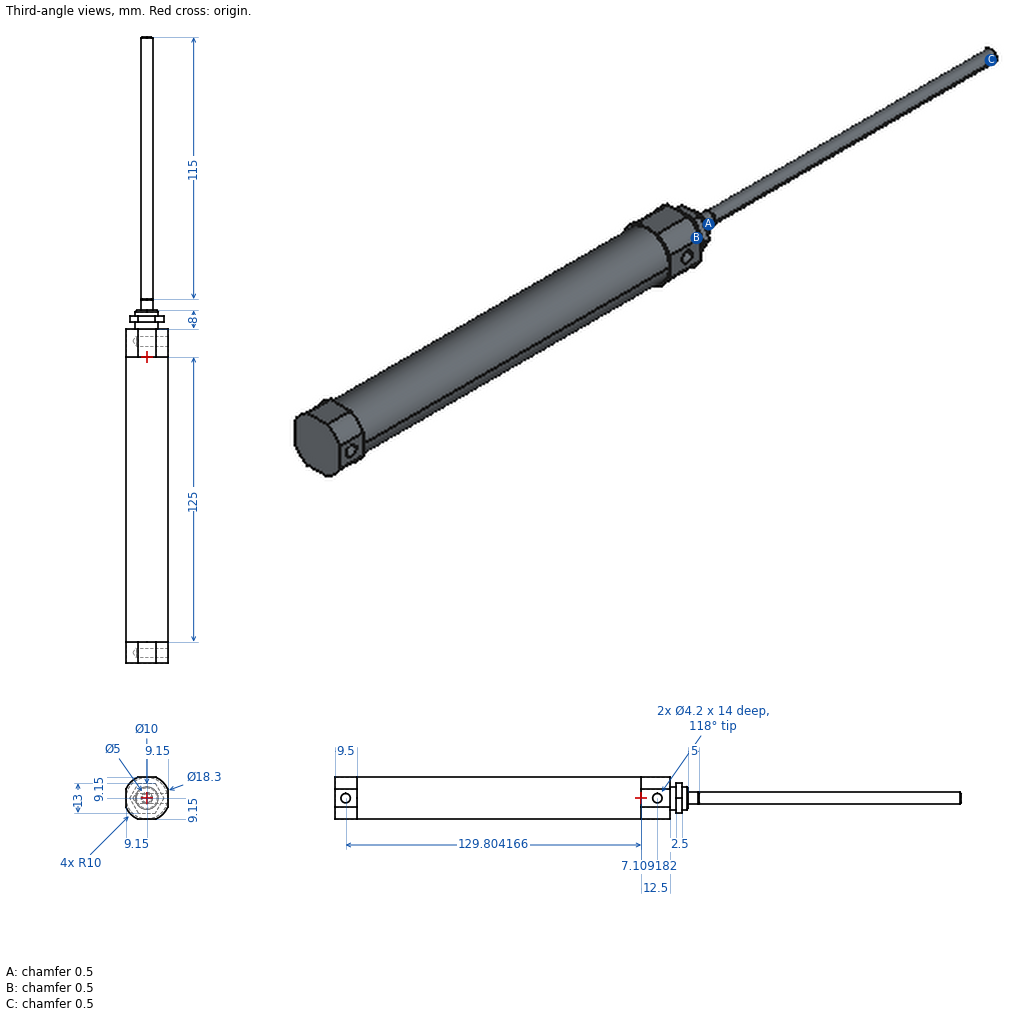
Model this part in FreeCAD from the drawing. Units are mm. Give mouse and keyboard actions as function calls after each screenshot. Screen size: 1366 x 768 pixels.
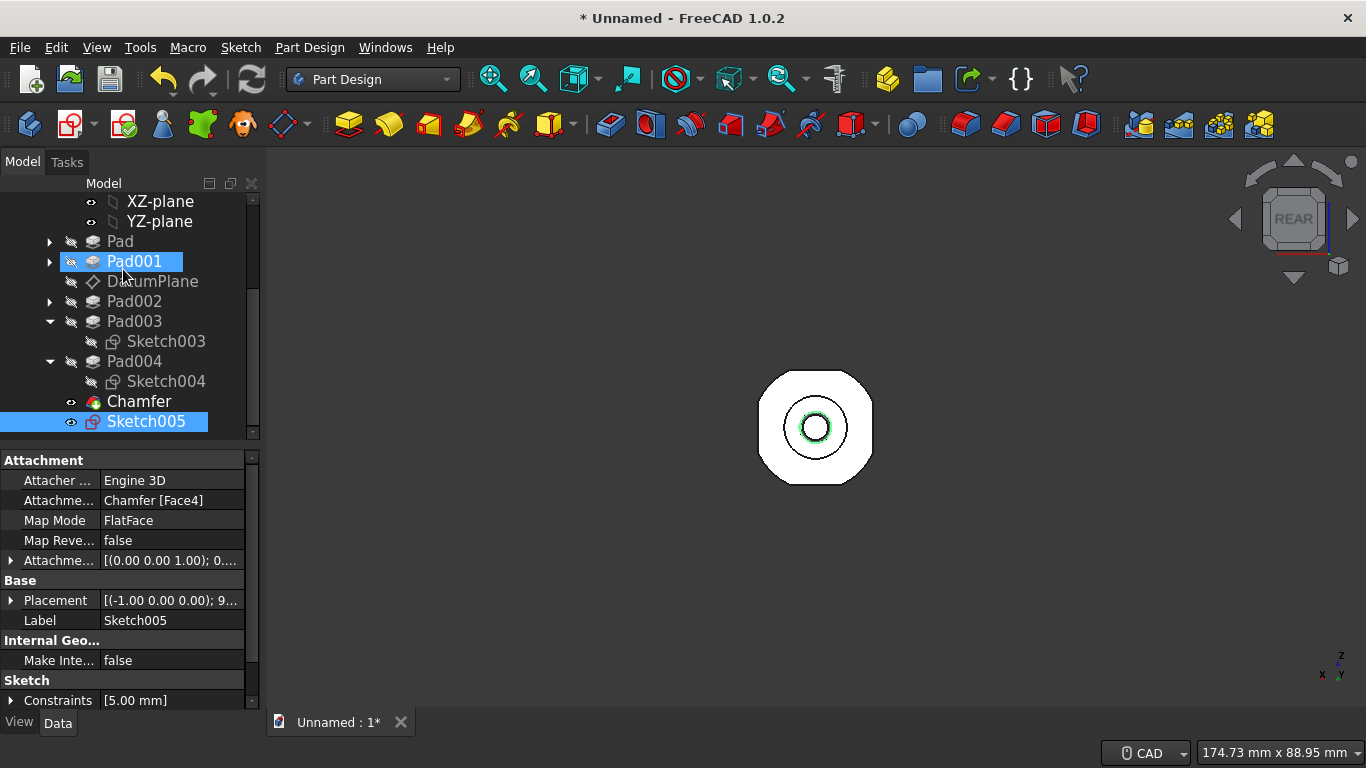
click(350, 124)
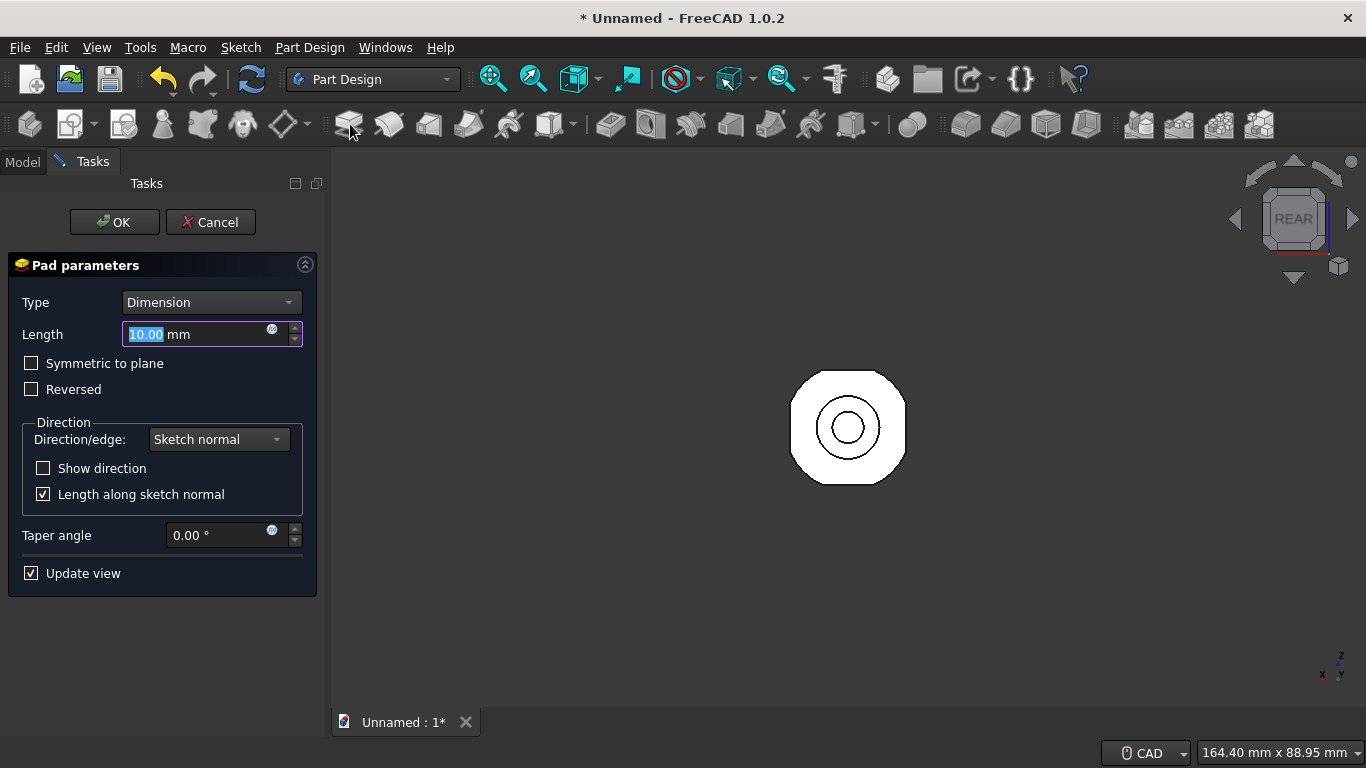
text(115)
key(Tab)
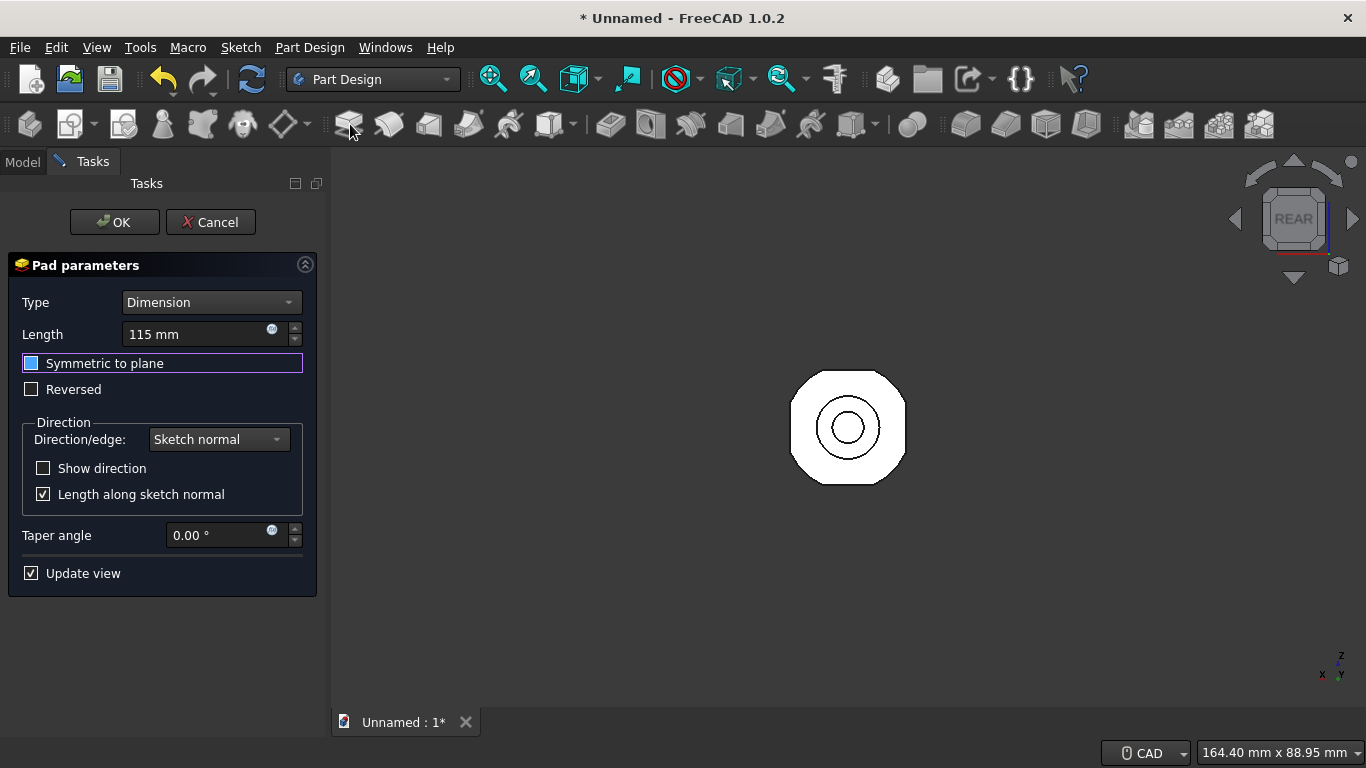
click(115, 222)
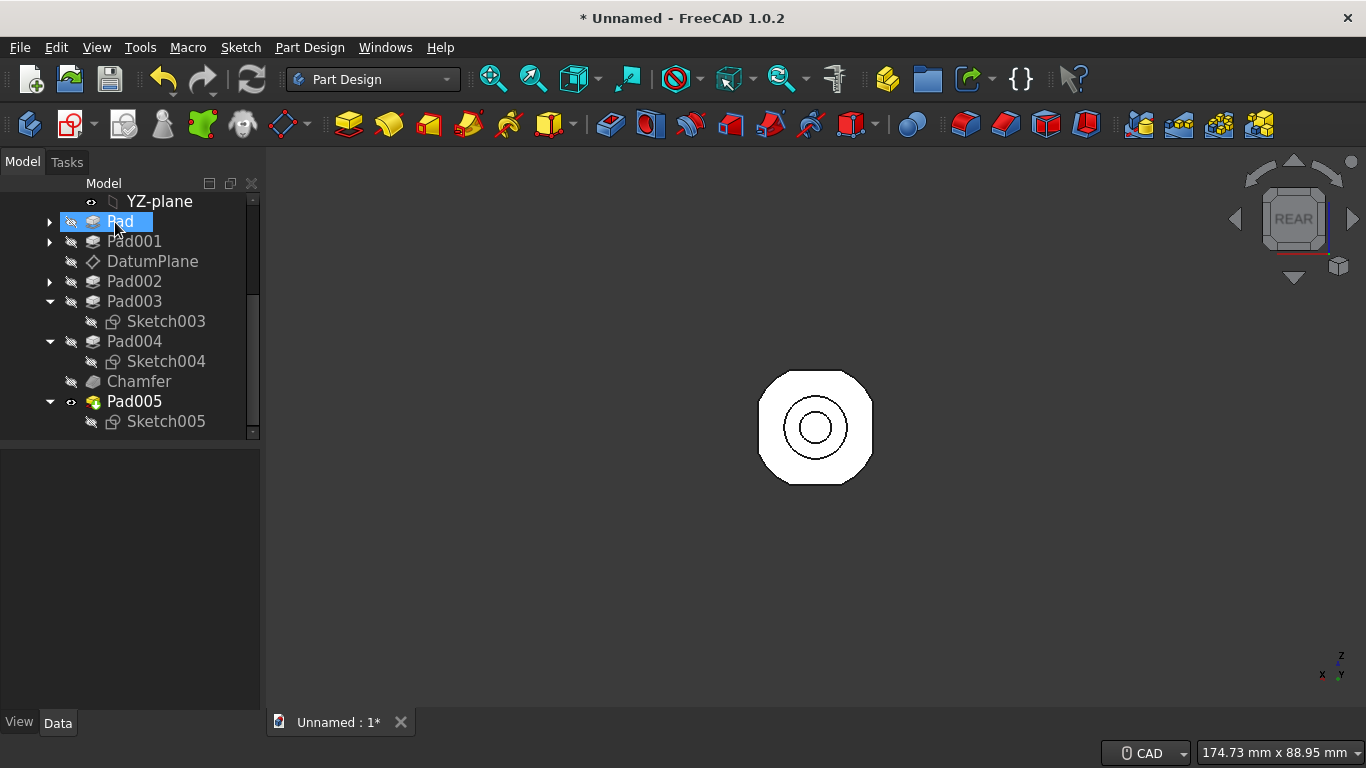
key(v)
key(f)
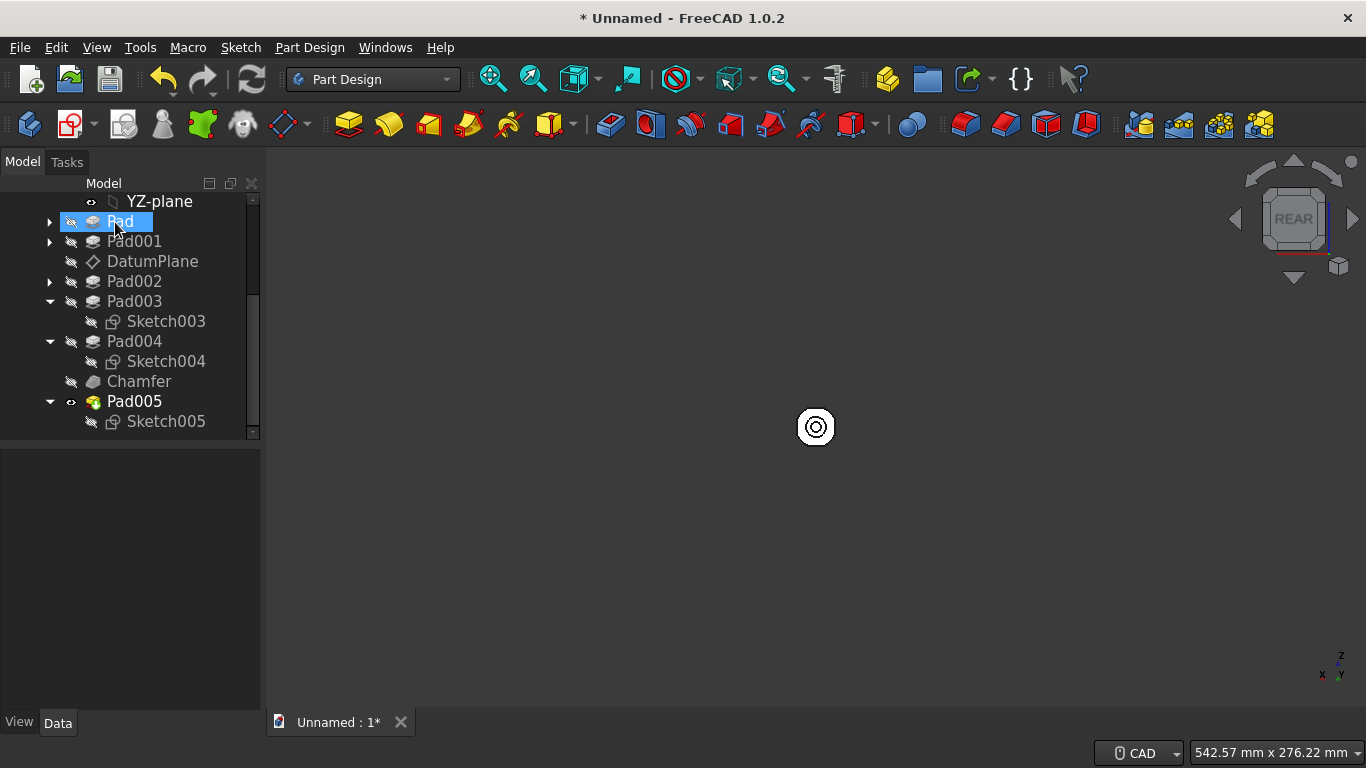
key(0)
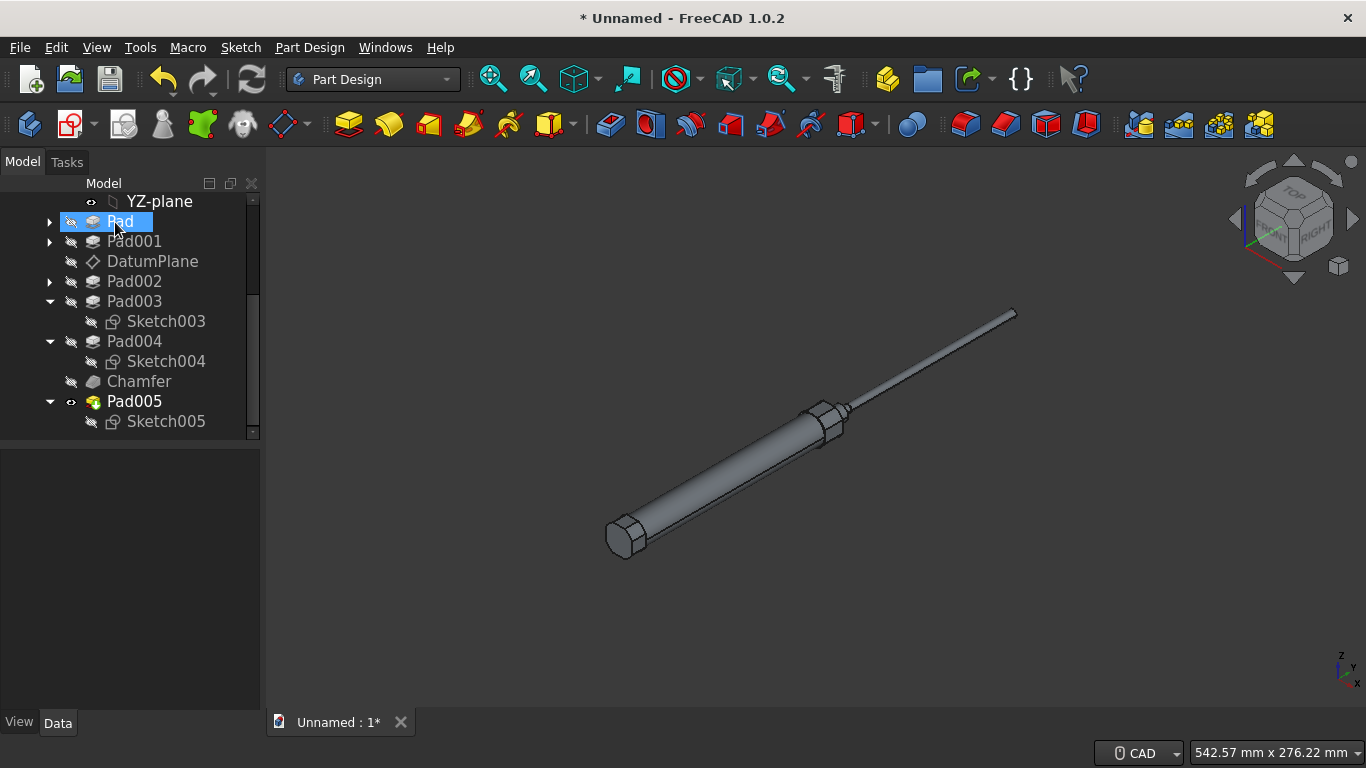
key(2)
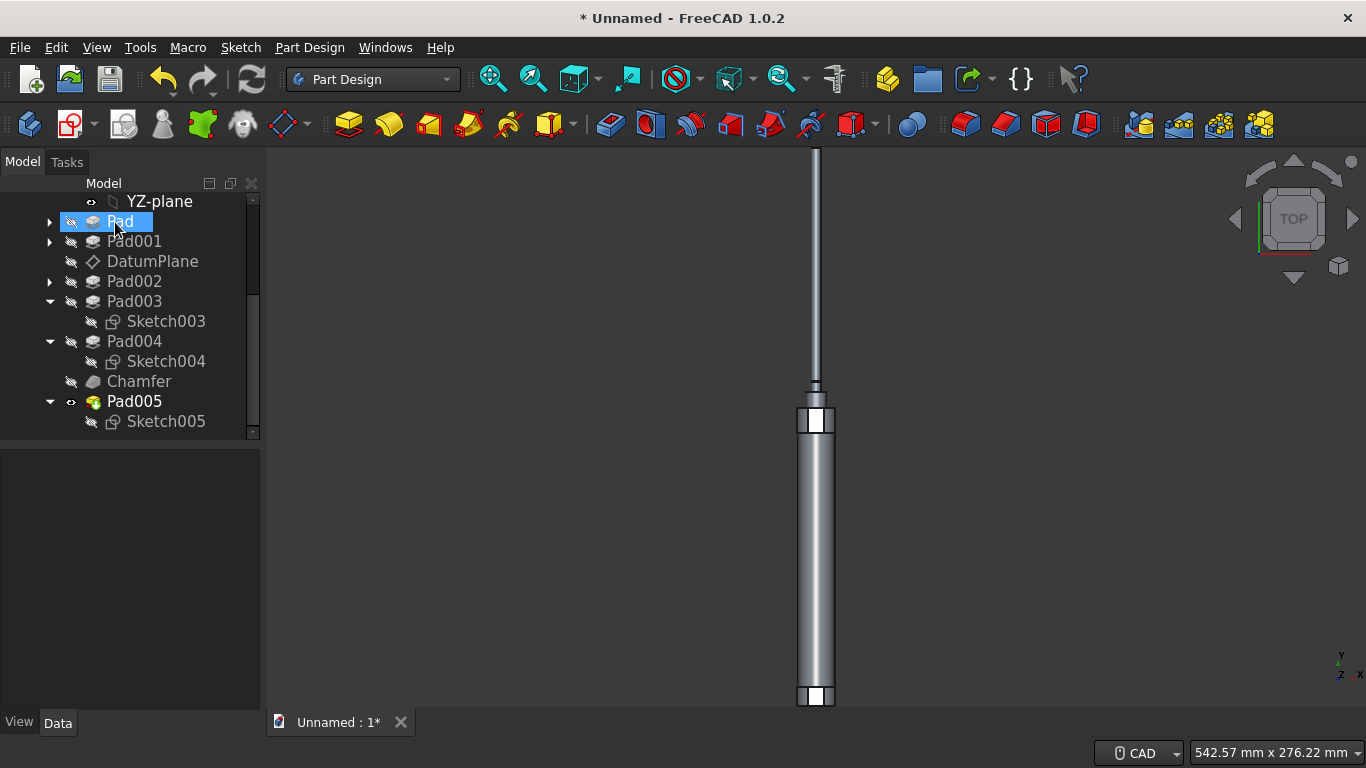
click(806, 391)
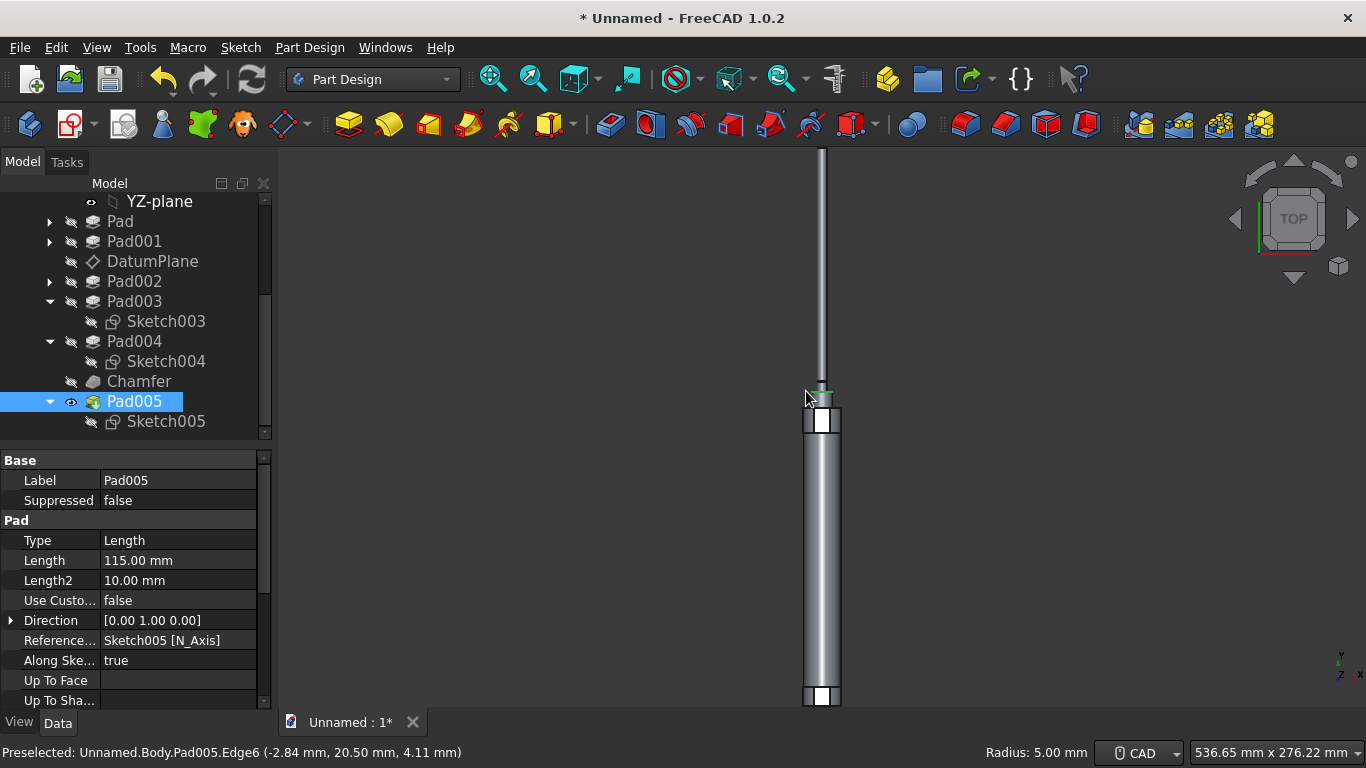
click(1006, 124)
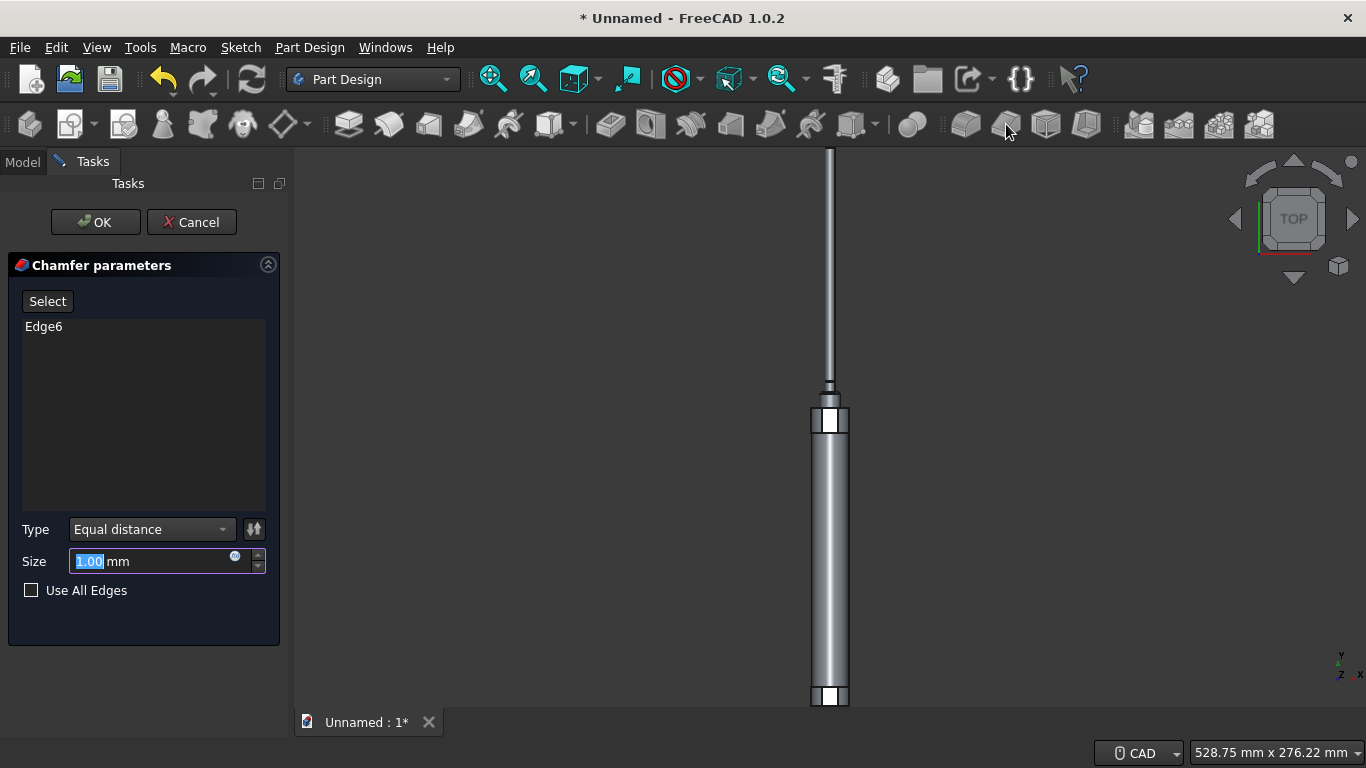
text(0.5)
key(Tab)